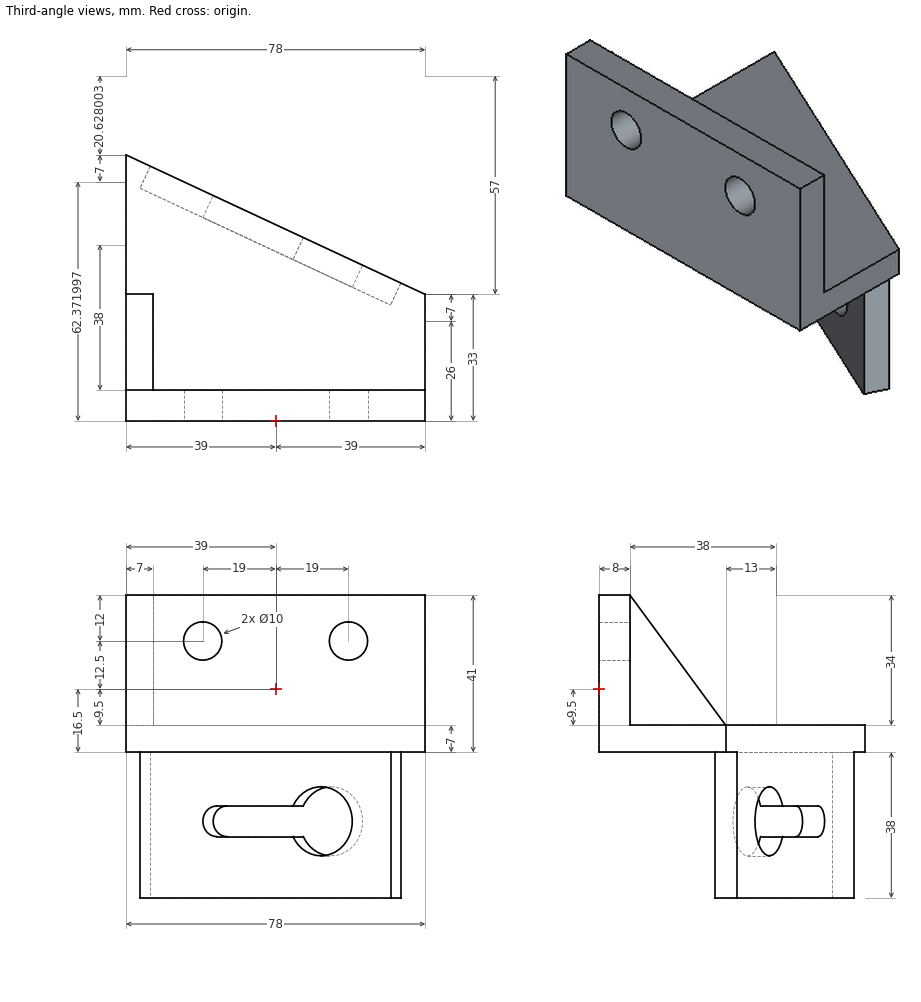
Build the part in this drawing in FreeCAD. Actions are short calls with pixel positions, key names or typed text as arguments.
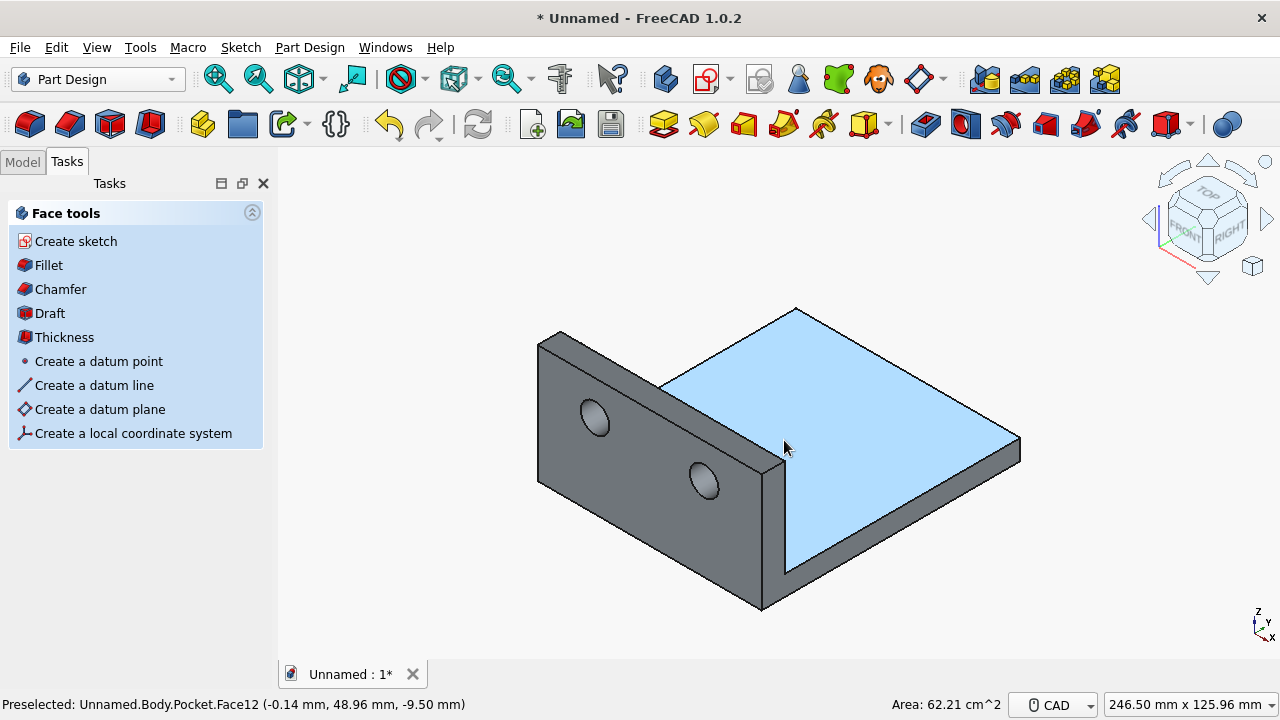
click(706, 80)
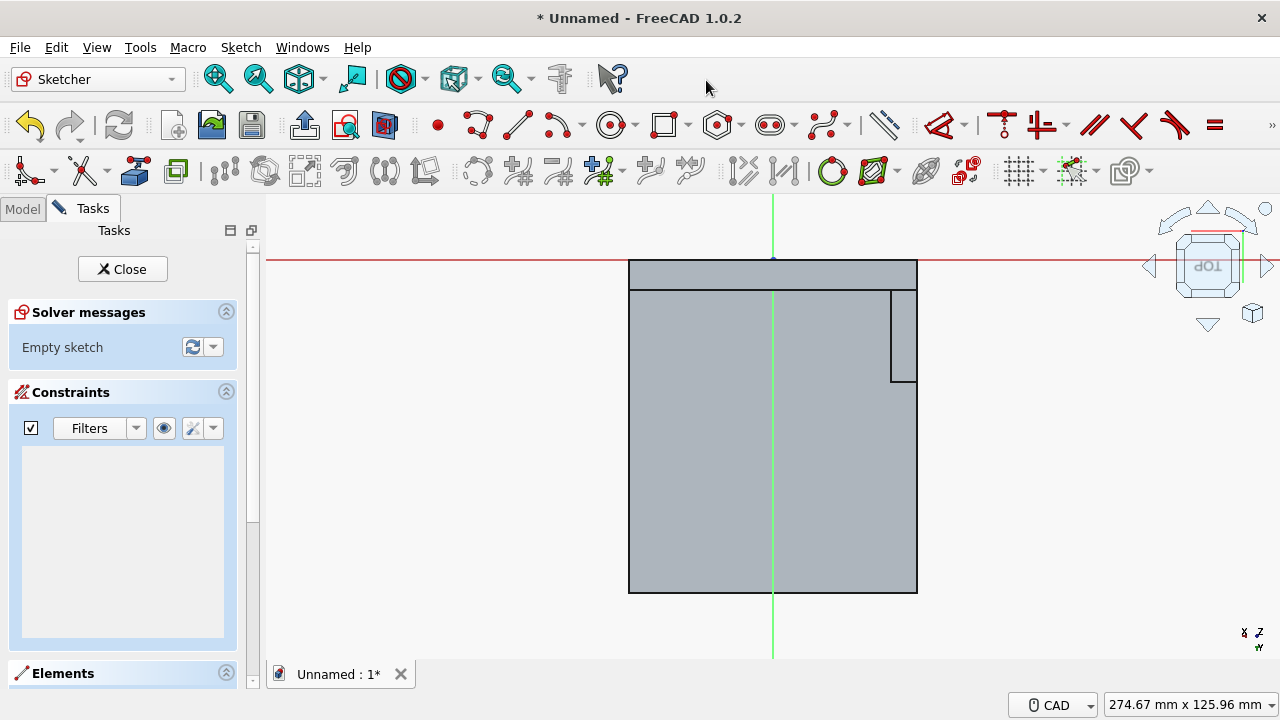
click(478, 126)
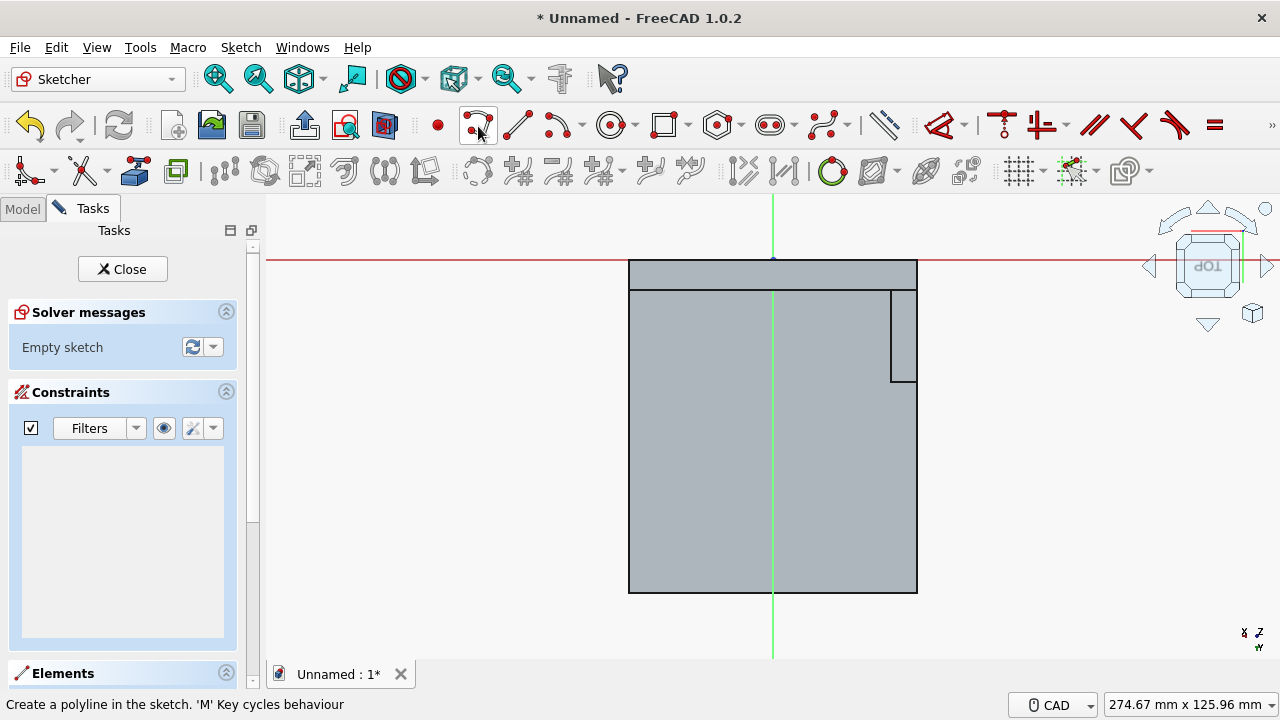
click(629, 382)
click(629, 593)
click(917, 593)
click(917, 516)
click(629, 383)
key(Escape)
key(Escape)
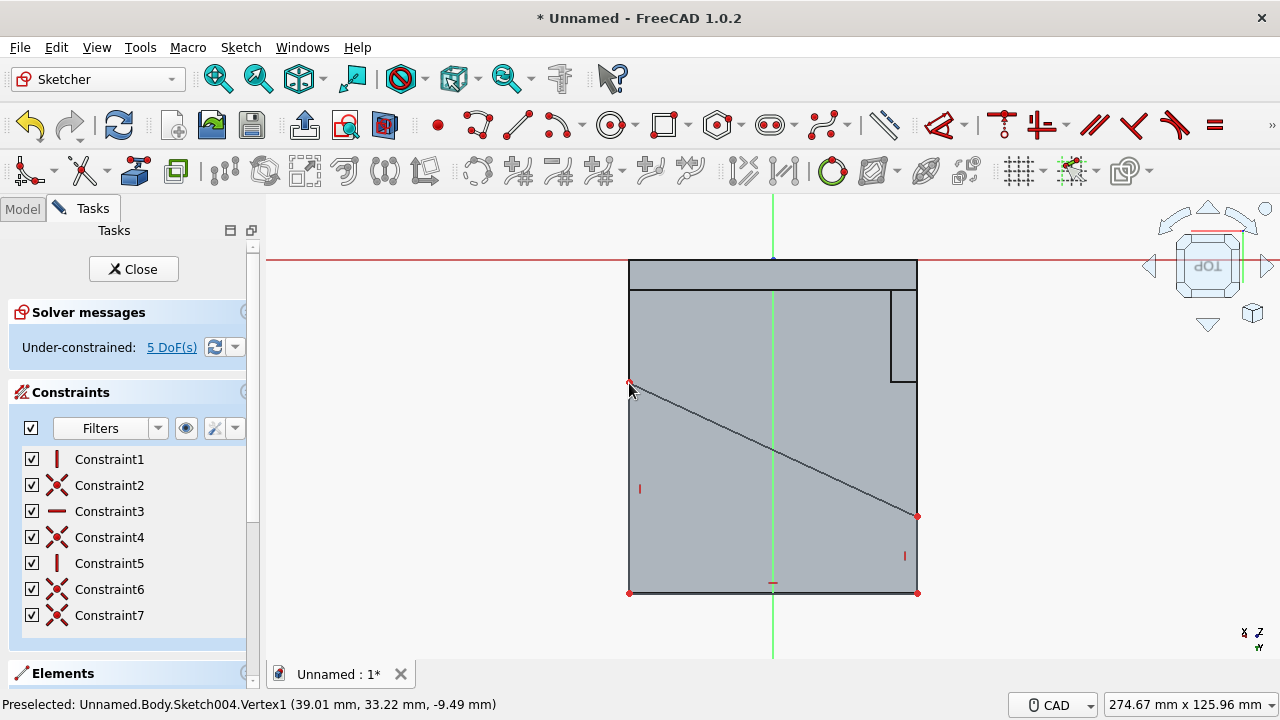
key(d)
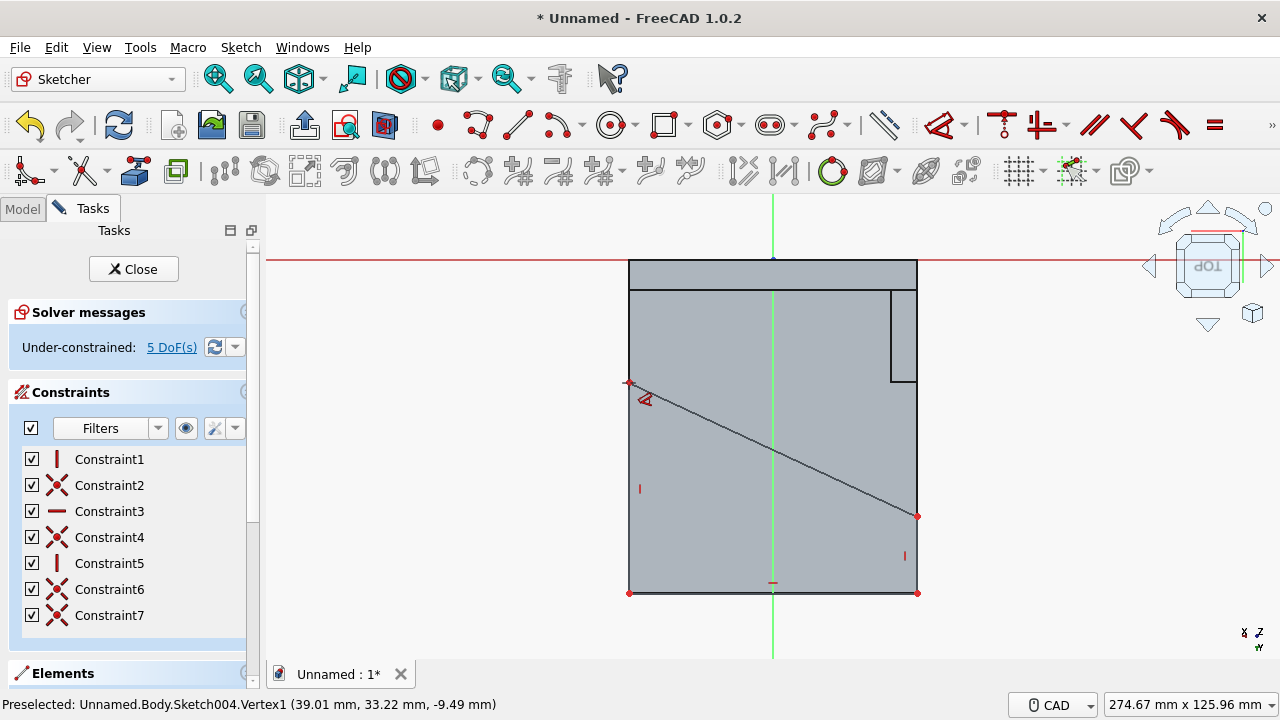
click(629, 446)
click(595, 489)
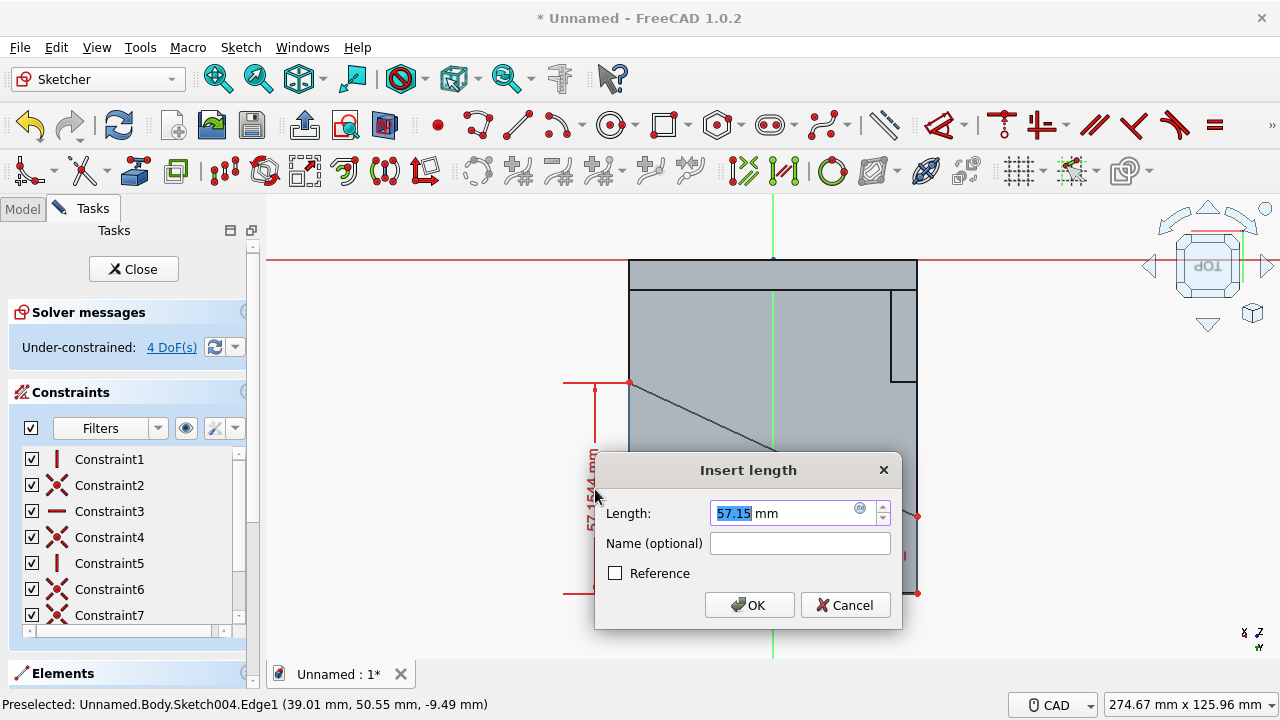
text(57)
key(Return)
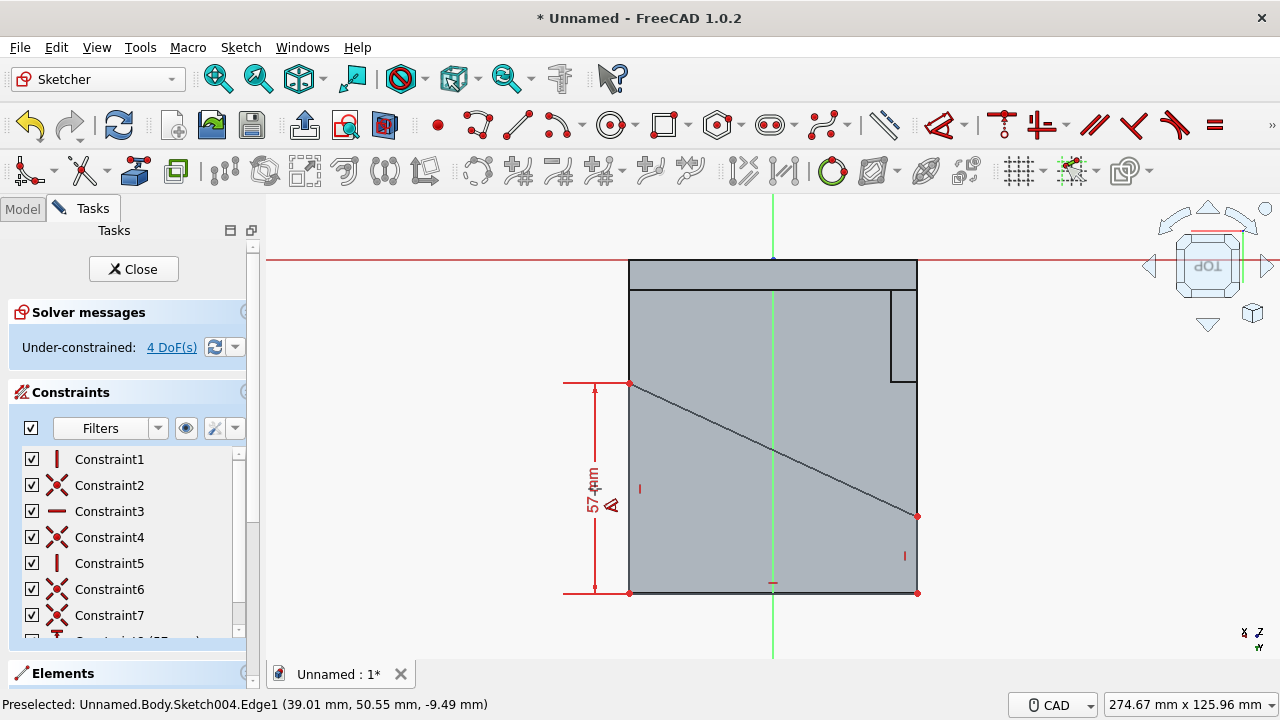
click(715, 594)
click(707, 628)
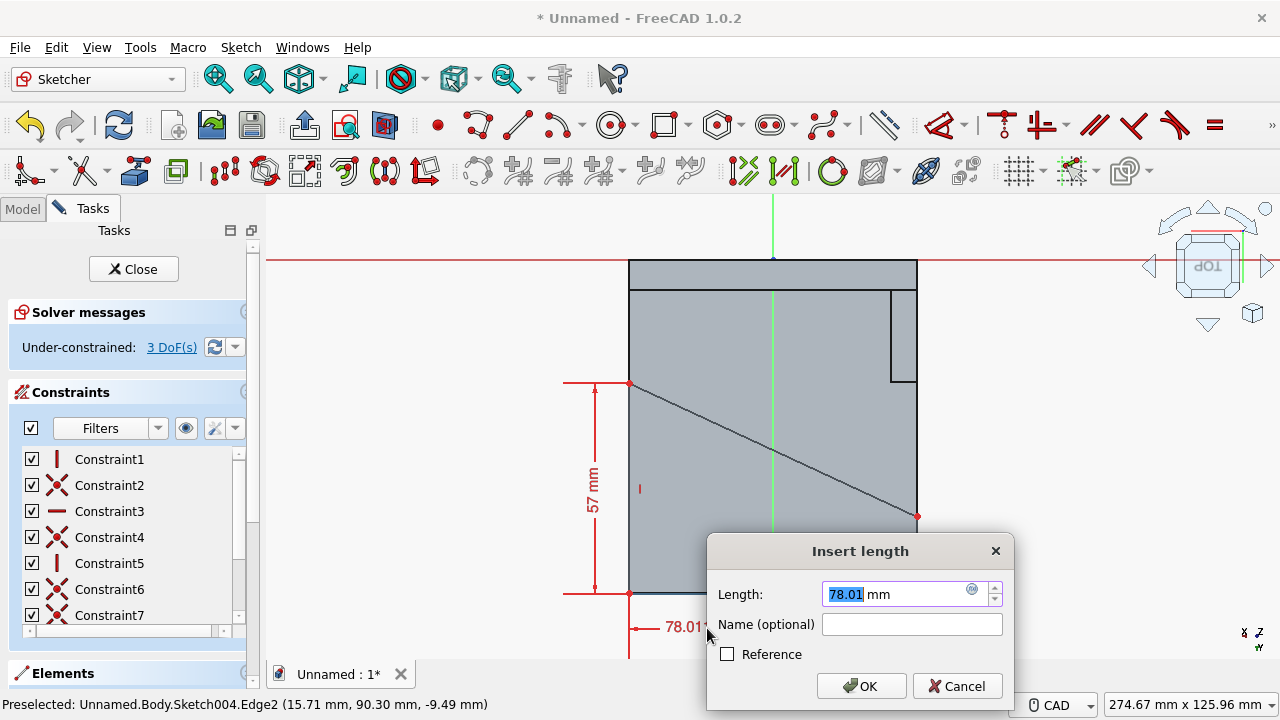
text(78)
key(Return)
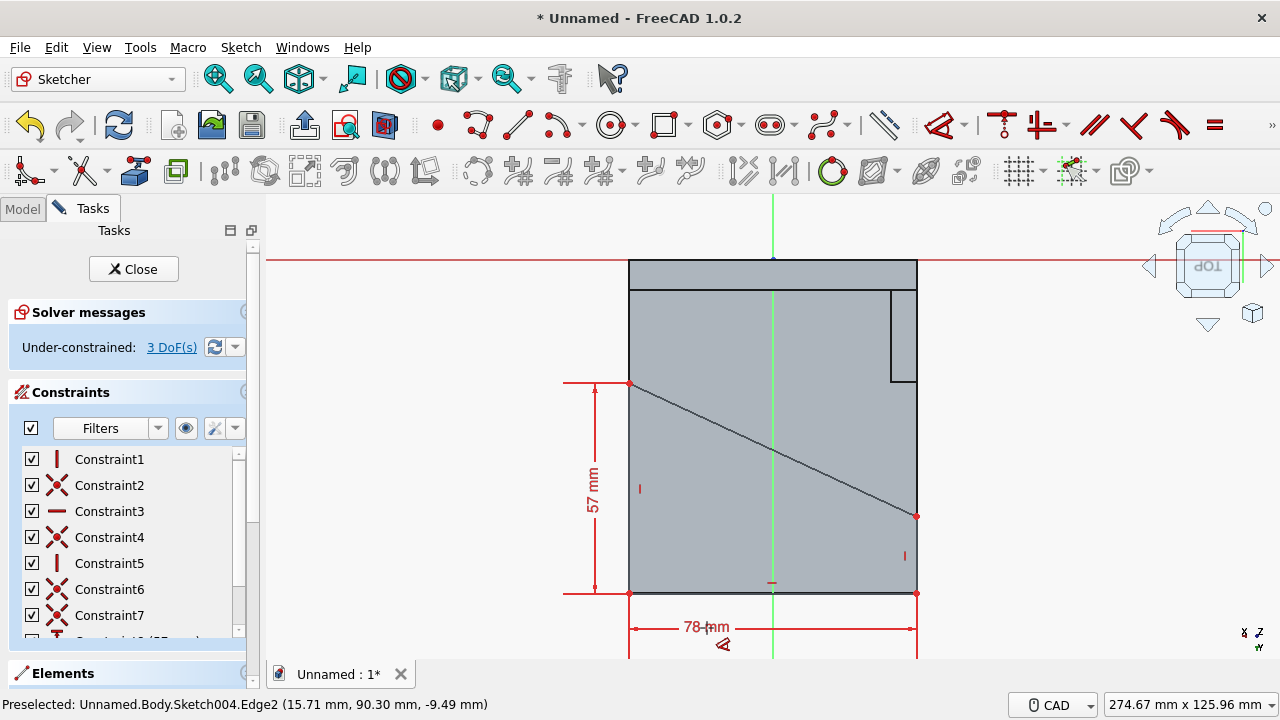
click(629, 383)
click(701, 226)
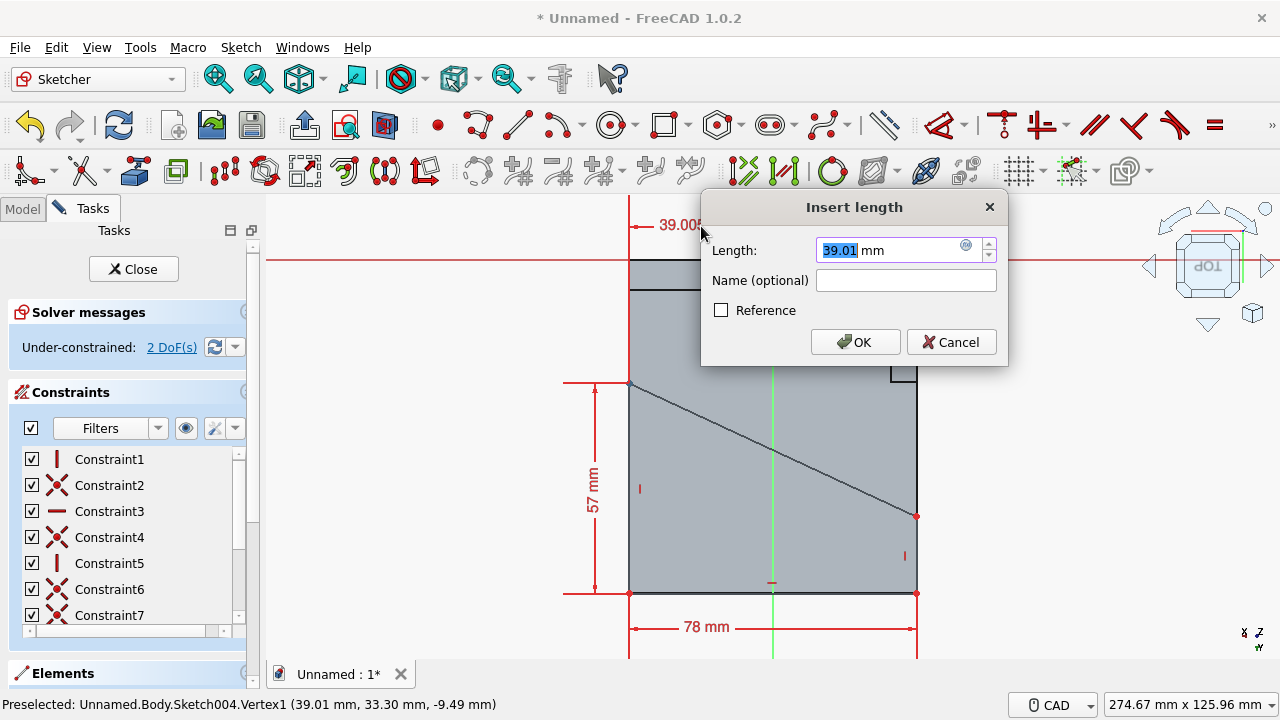
text(39)
key(Return)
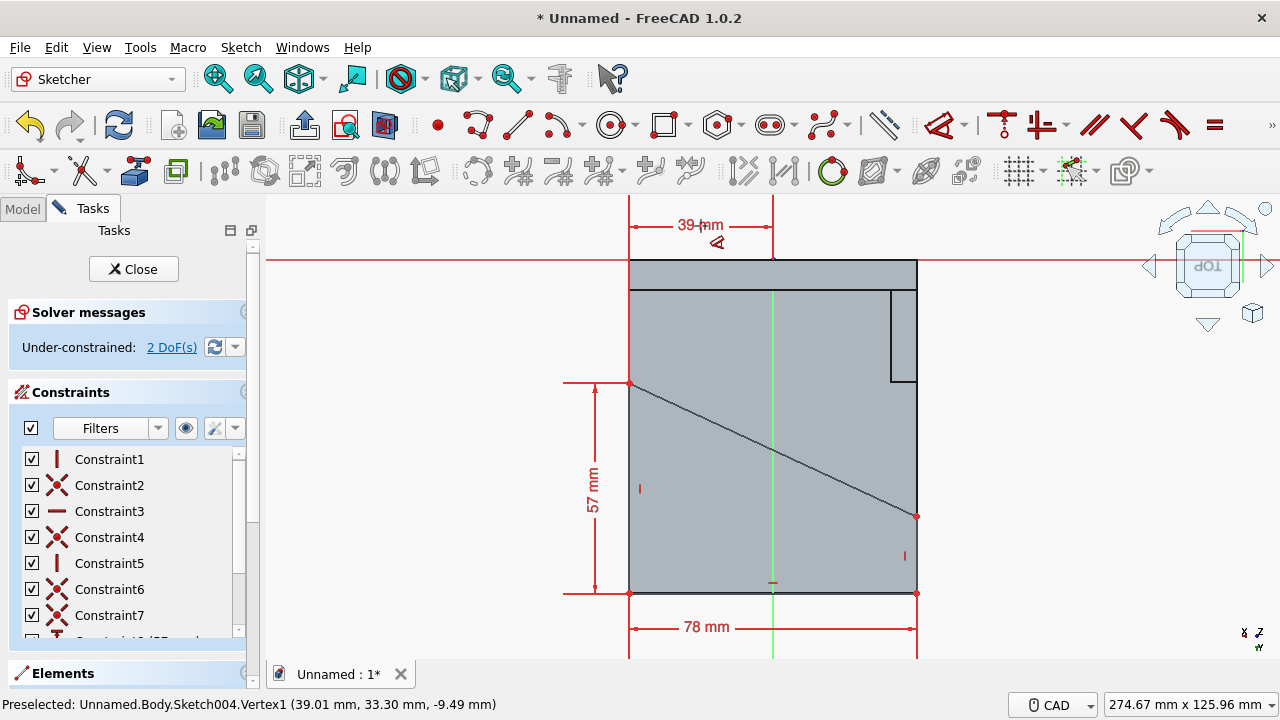
click(629, 383)
click(595, 322)